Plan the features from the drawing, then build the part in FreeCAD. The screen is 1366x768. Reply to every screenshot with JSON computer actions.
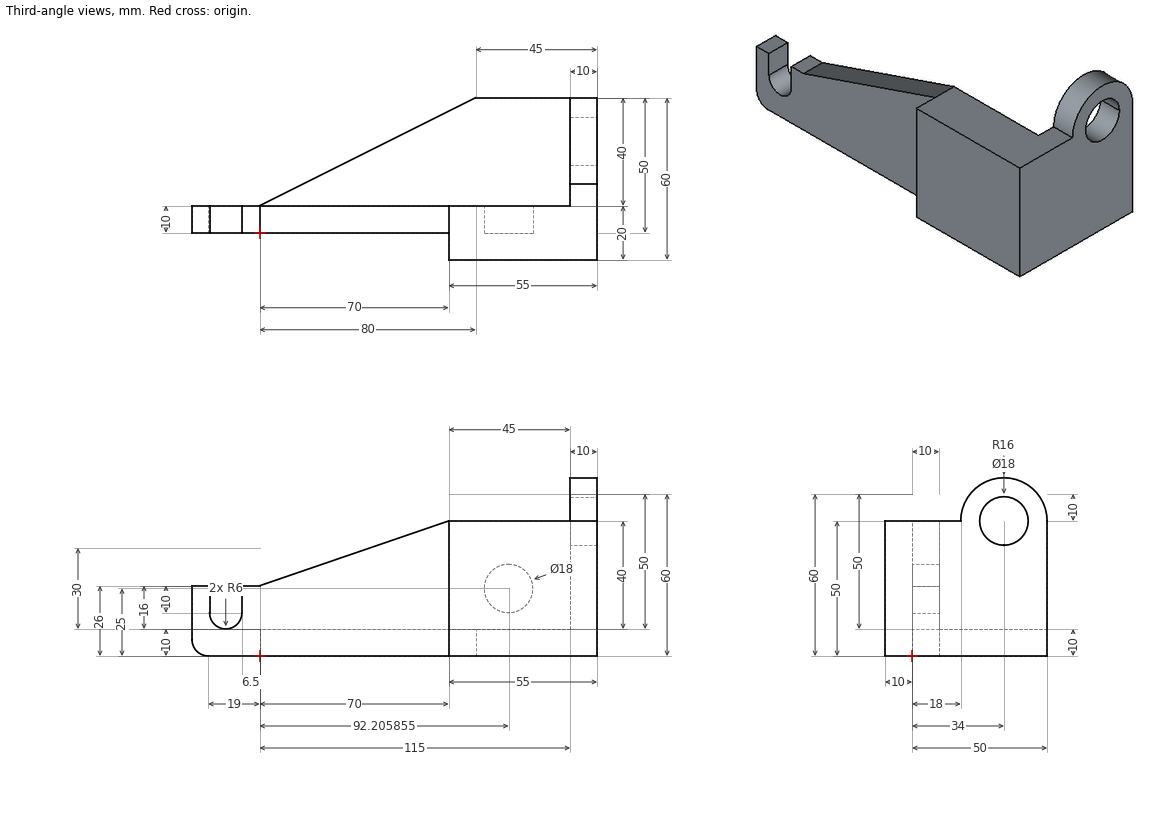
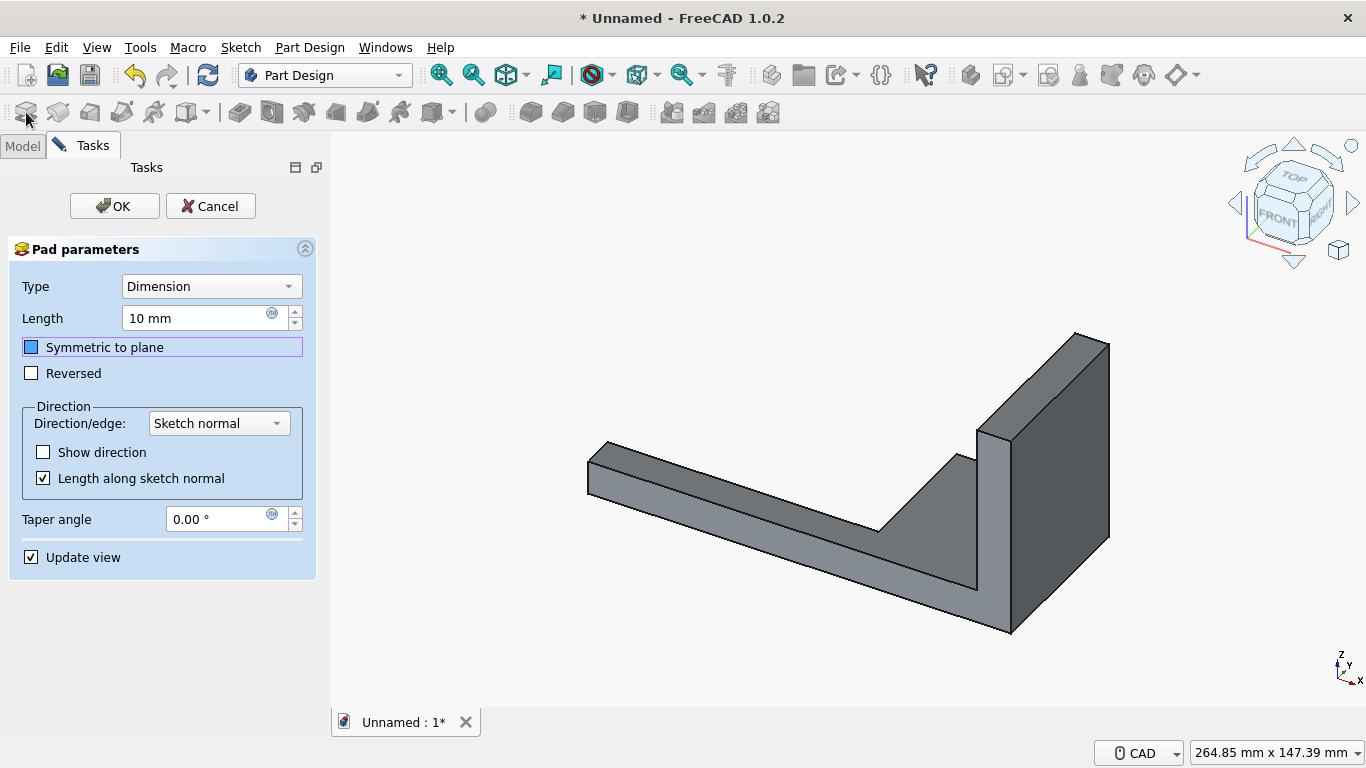
{"action": "left_click", "coordinate": [30, 373]}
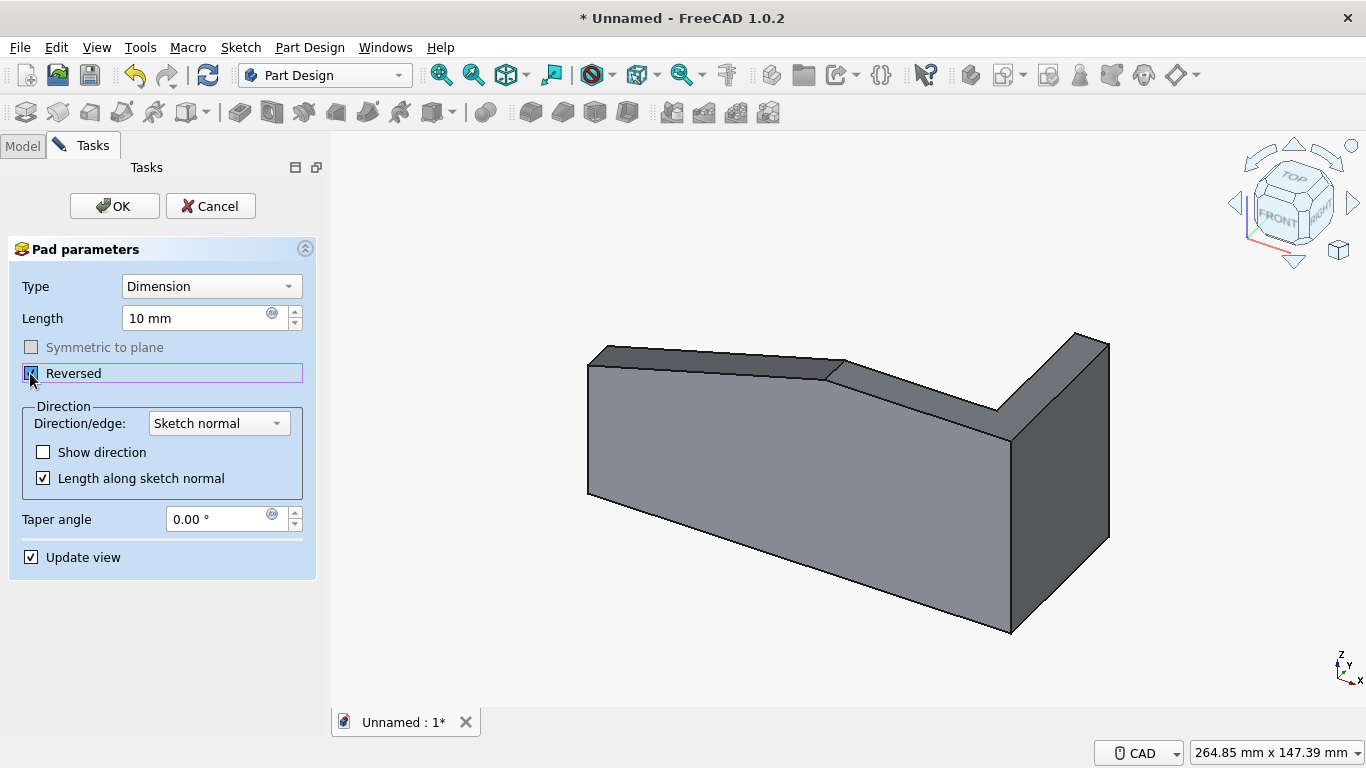
{"action": "left_click", "coordinate": [115, 206]}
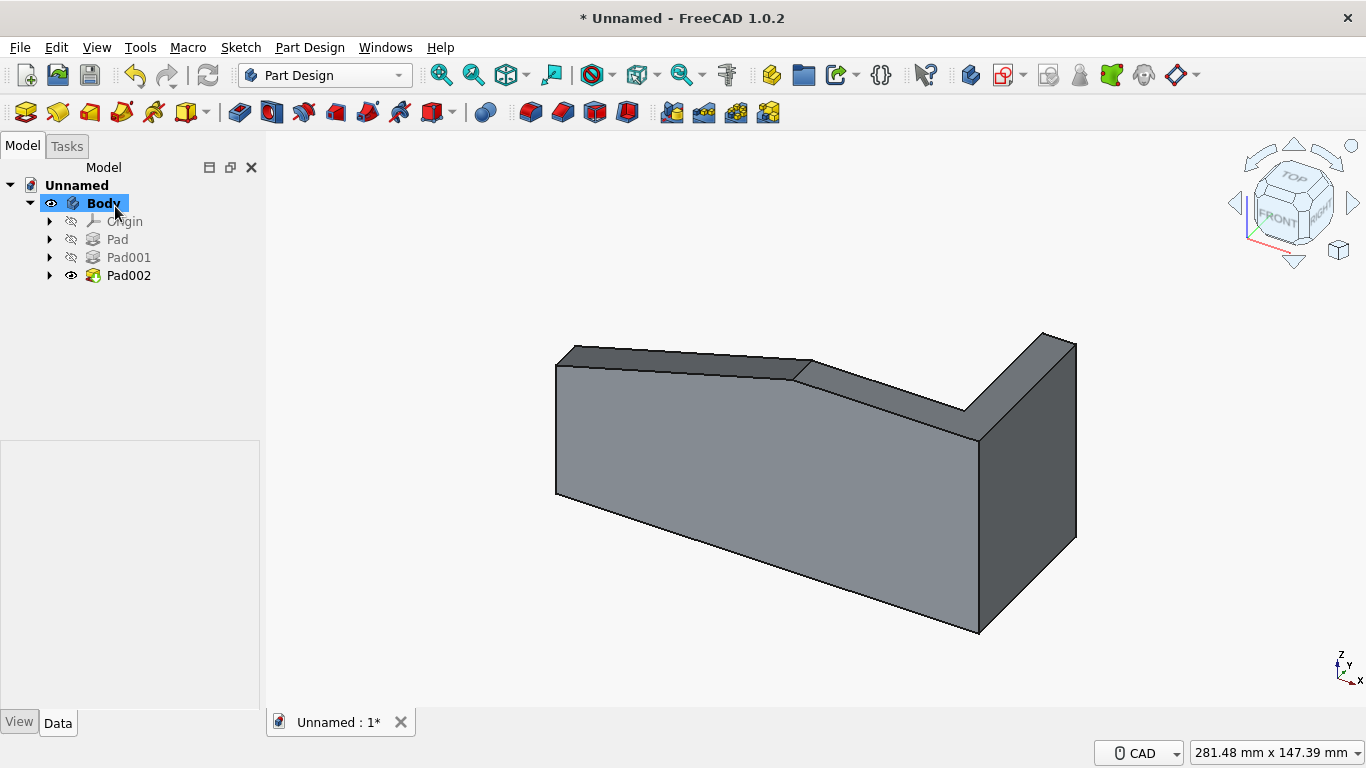
{"action": "left_click", "coordinate": [1004, 76]}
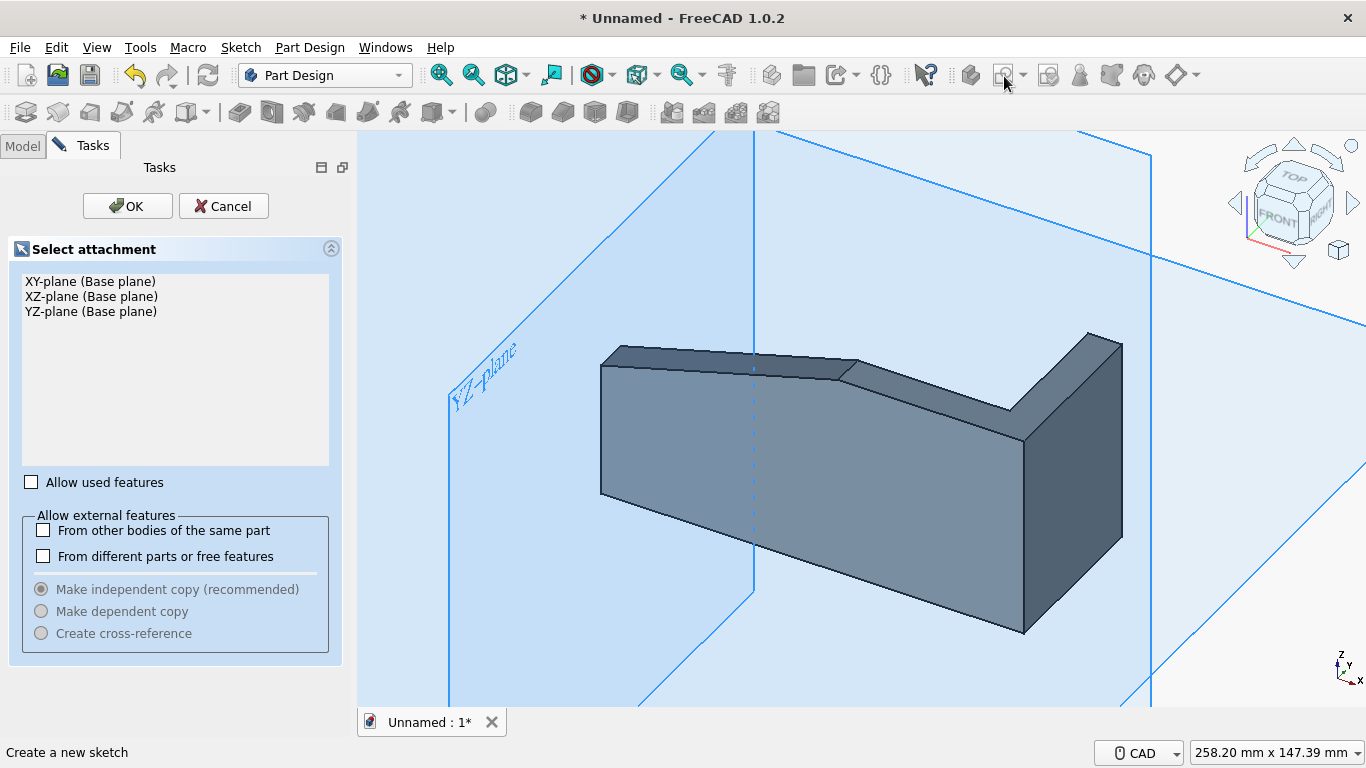
{"action": "left_click", "coordinate": [82, 282]}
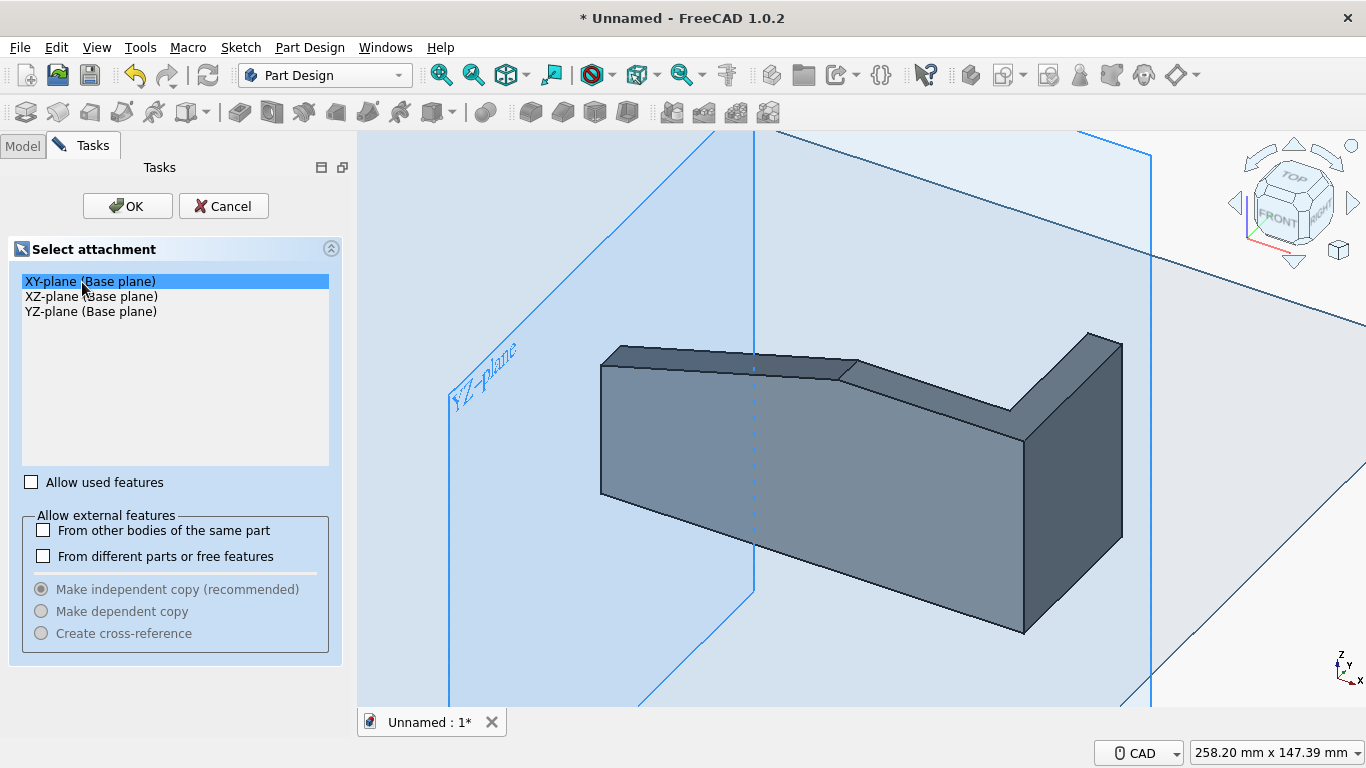
{"action": "left_click", "coordinate": [128, 206]}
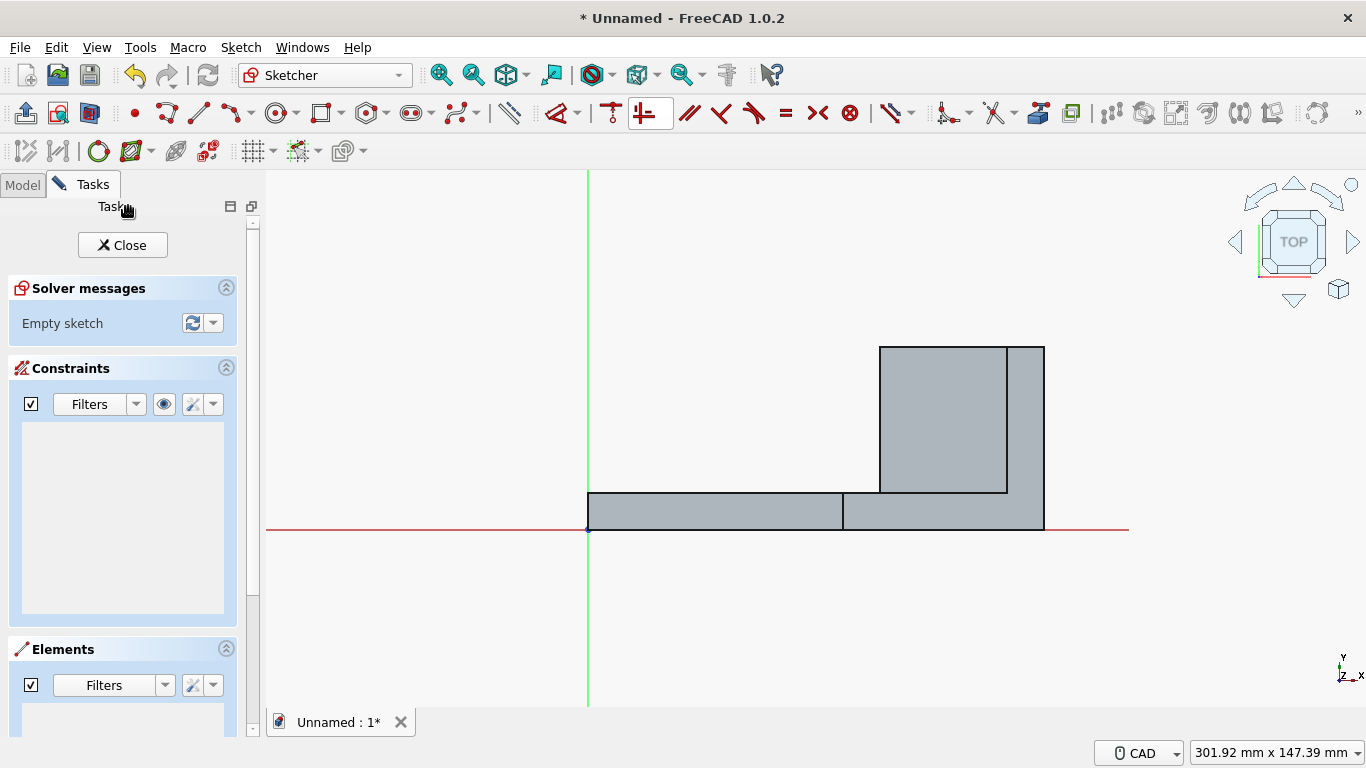
{"action": "left_click", "coordinate": [90, 114]}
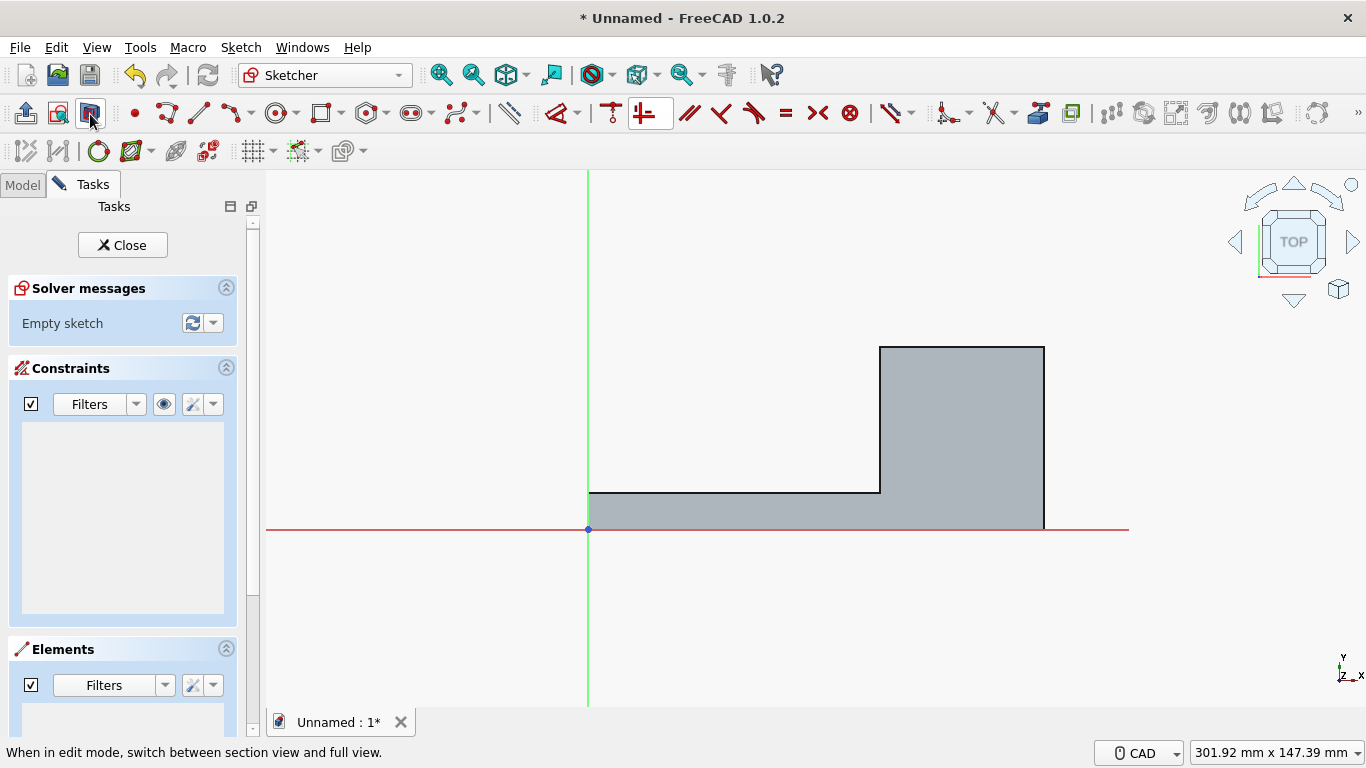
{"action": "scroll", "coordinate": [718, 438], "scroll_direction": "up", "scroll_amount": 3}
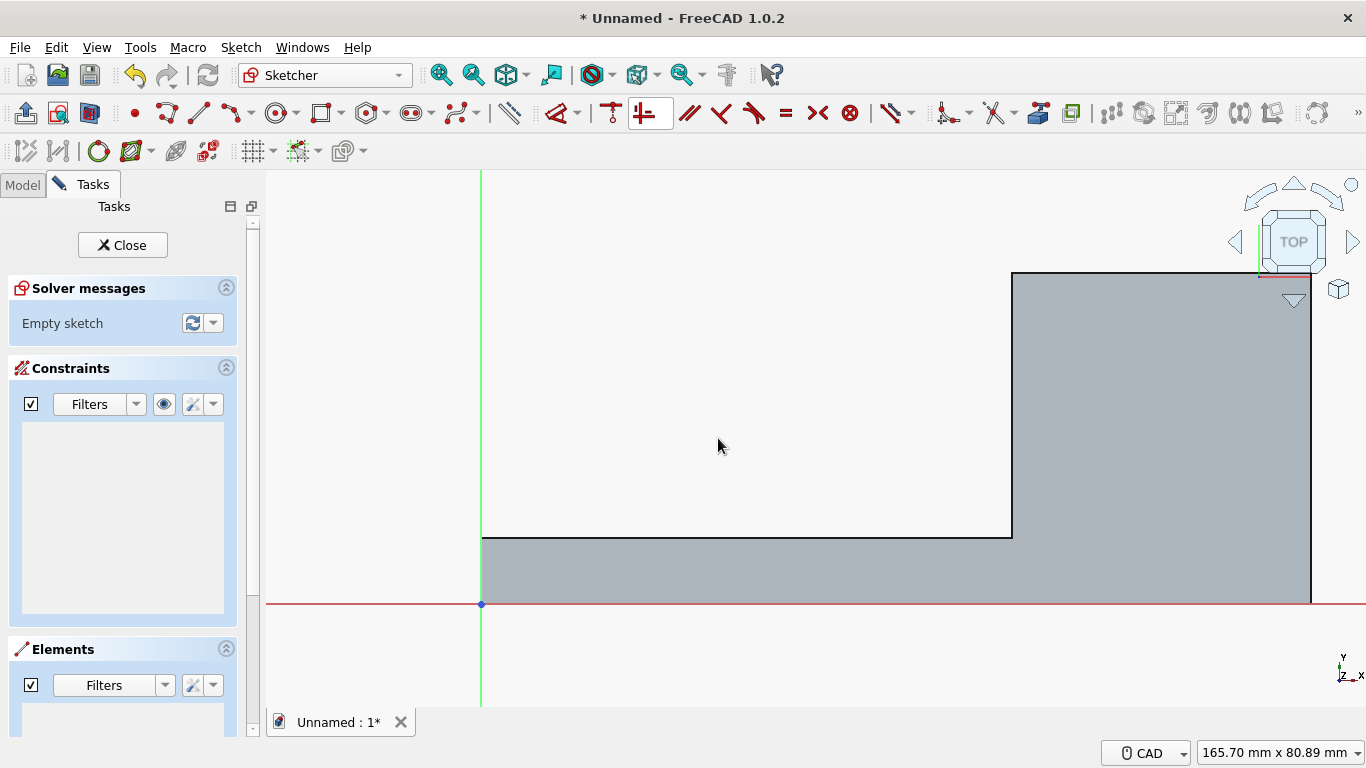
{"action": "left_click", "coordinate": [168, 114]}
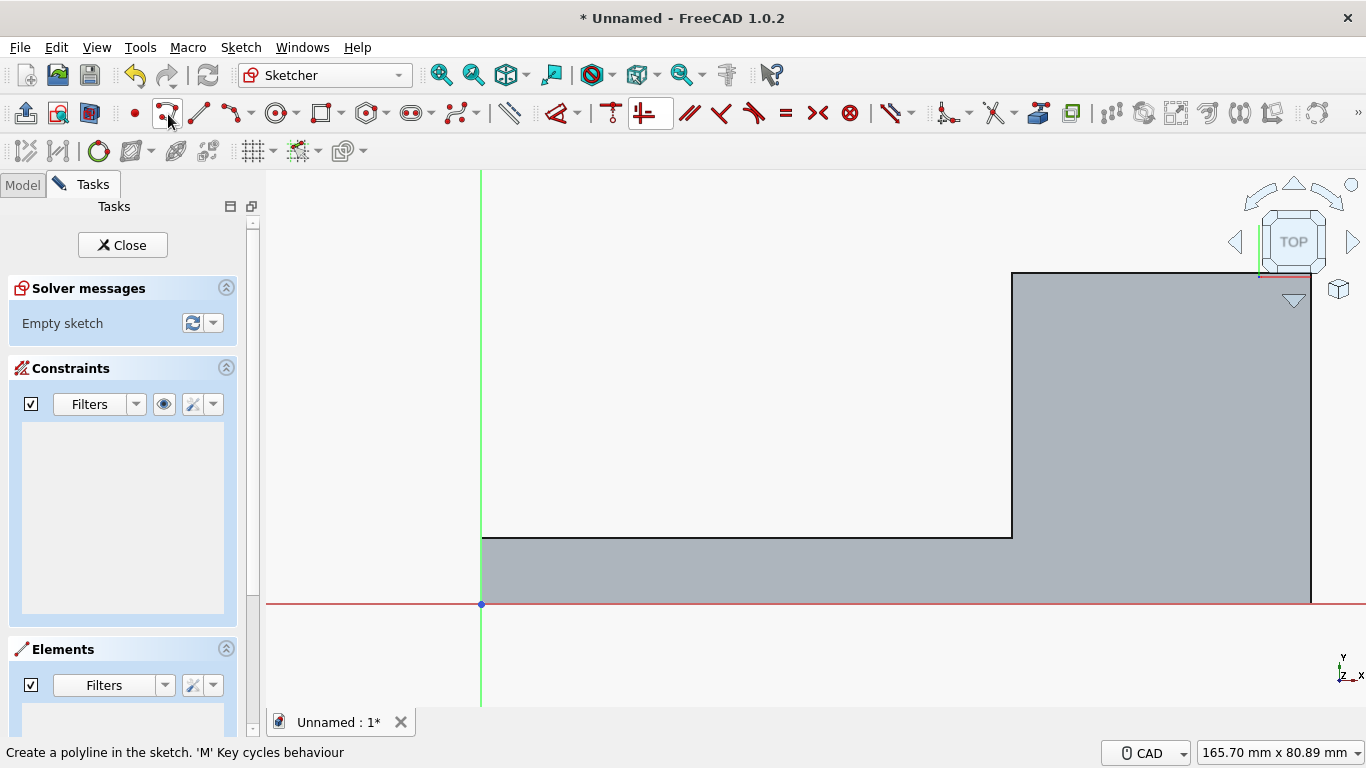
{"action": "left_click", "coordinate": [481, 538]}
{"action": "left_click", "coordinate": [1012, 273]}
{"action": "left_click", "coordinate": [1012, 538]}
{"action": "left_click", "coordinate": [481, 539]}
{"action": "key", "text": "Escape"}
{"action": "key", "text": "Escape"}